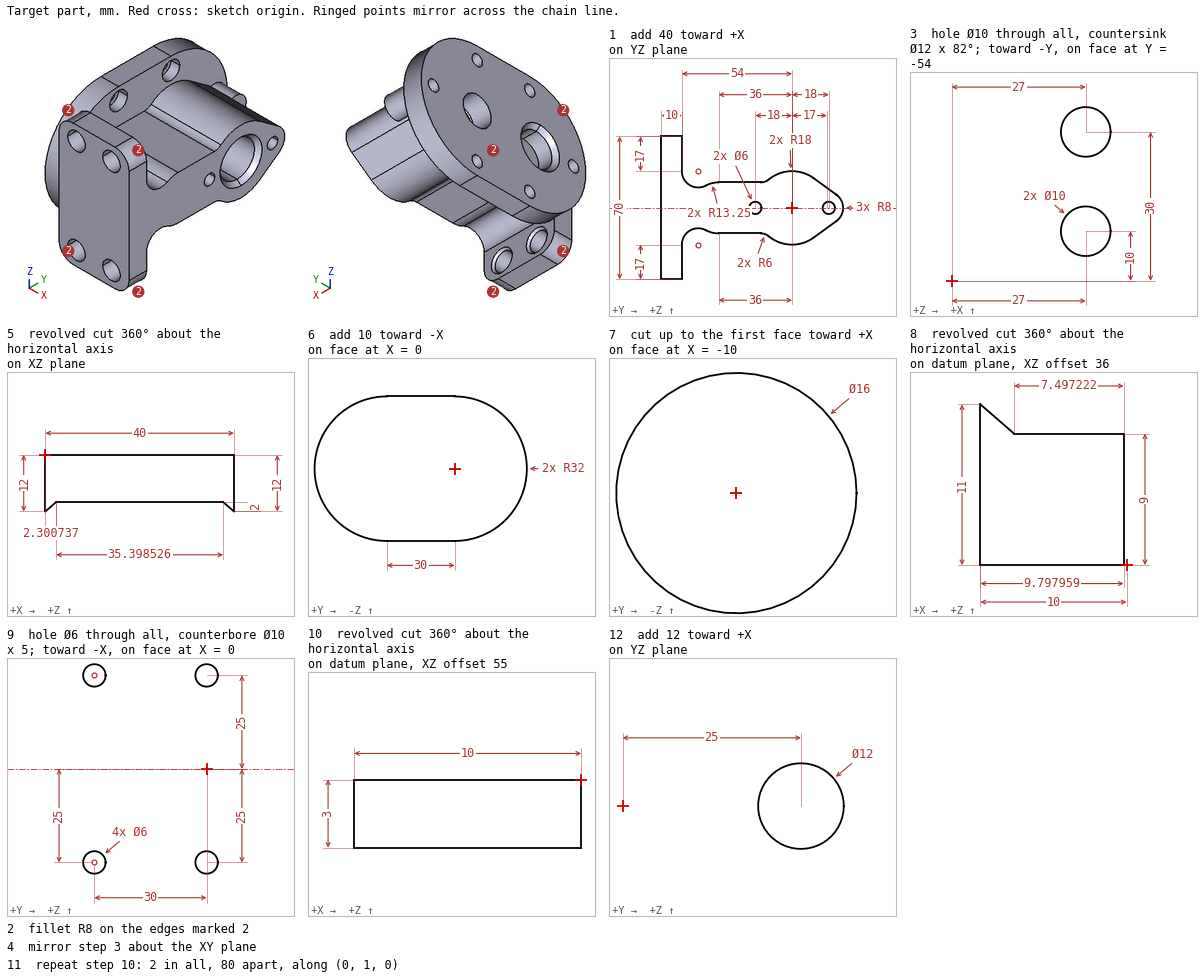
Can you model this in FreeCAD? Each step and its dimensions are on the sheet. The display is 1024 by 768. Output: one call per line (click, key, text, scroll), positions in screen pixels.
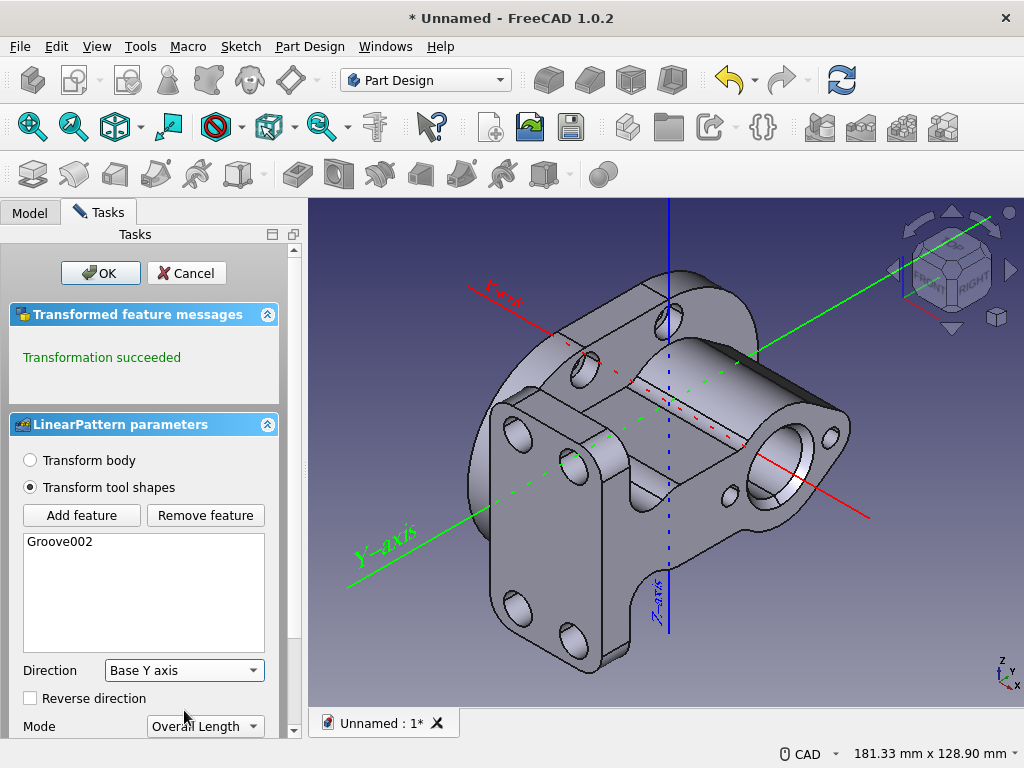
click(206, 726)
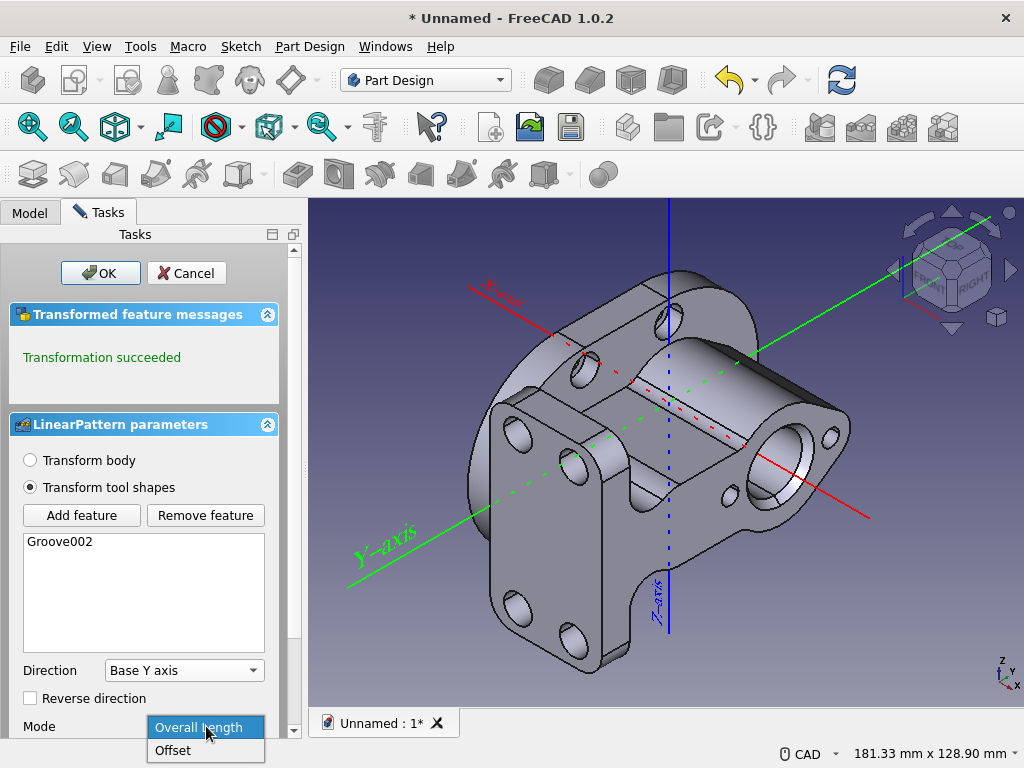
click(204, 750)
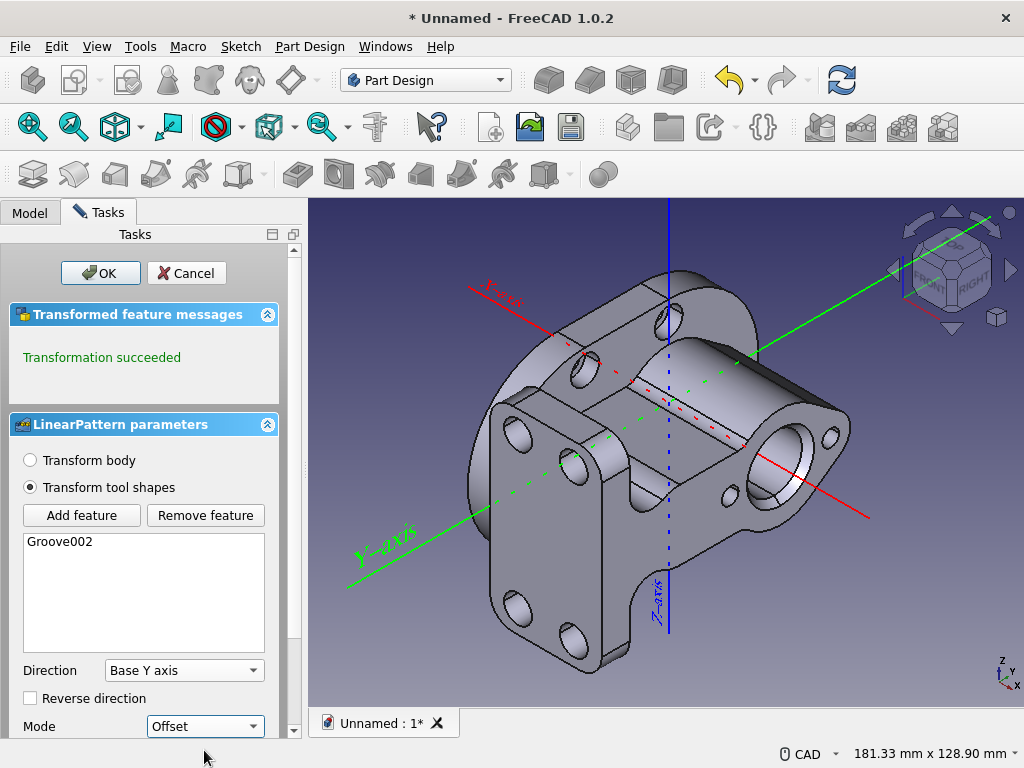
scroll(294, 491, down, 2)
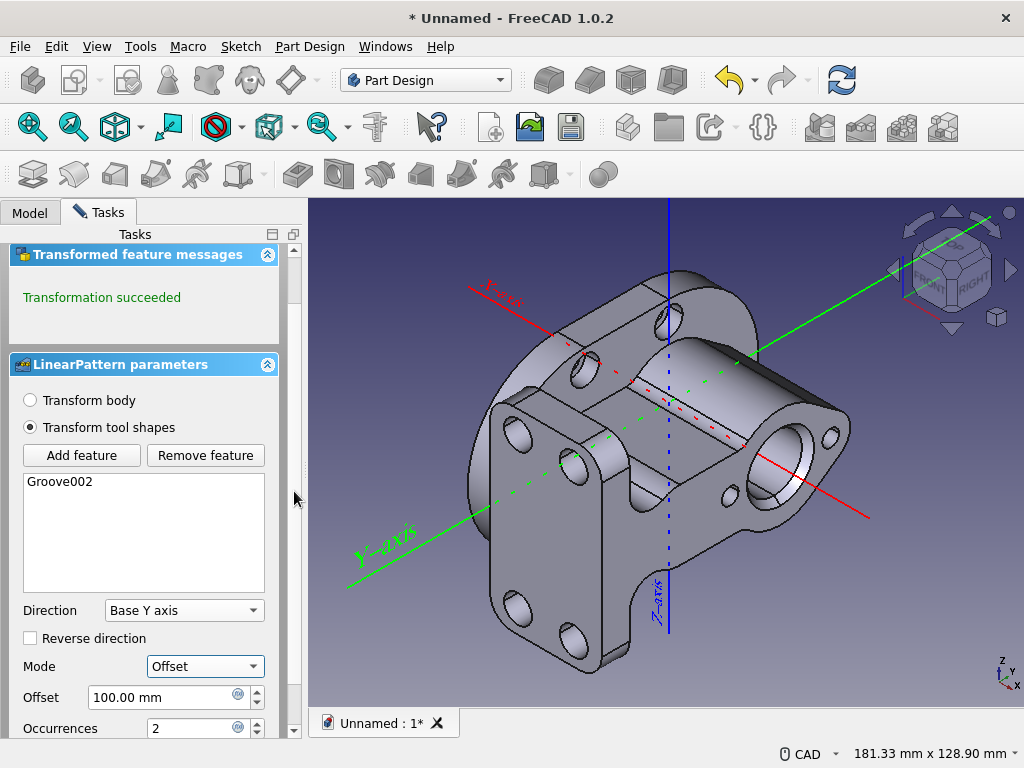
triple_click(170, 646)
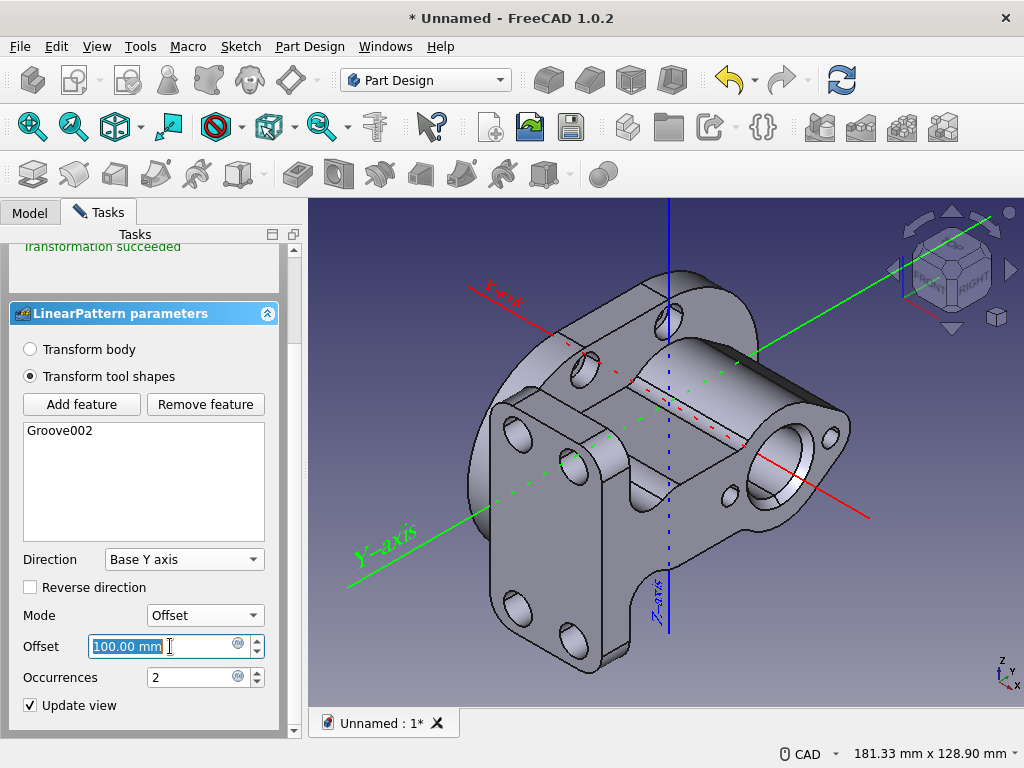
text(80)
key(Tab)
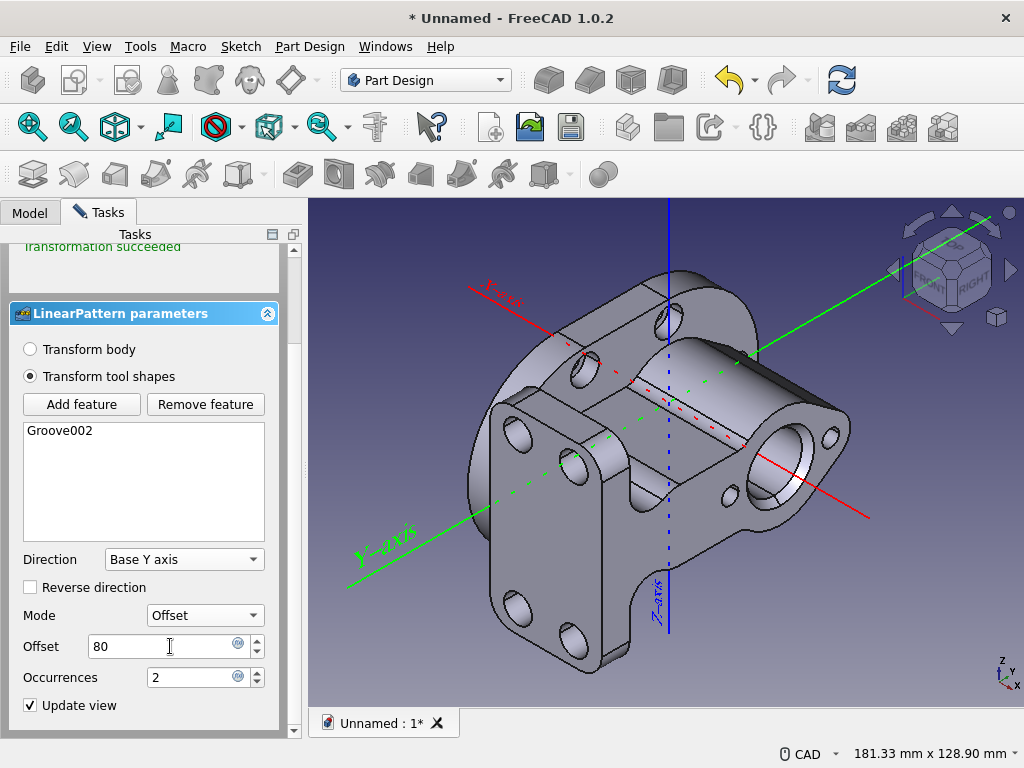
triple_click(199, 678)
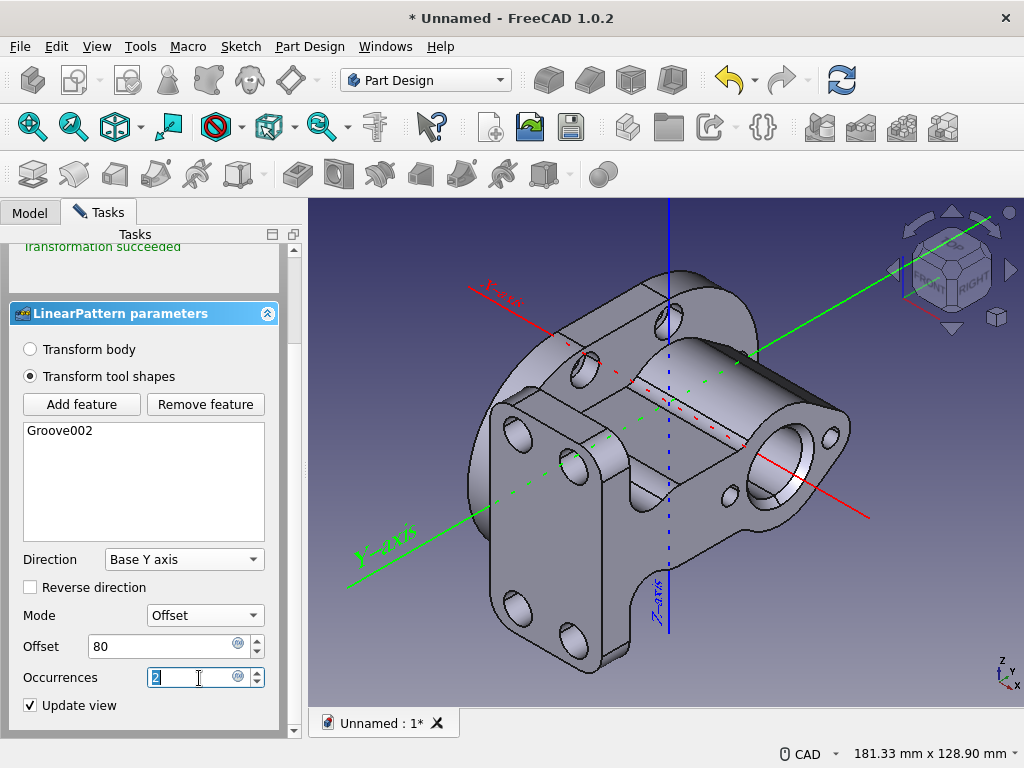
text(2)
key(Tab)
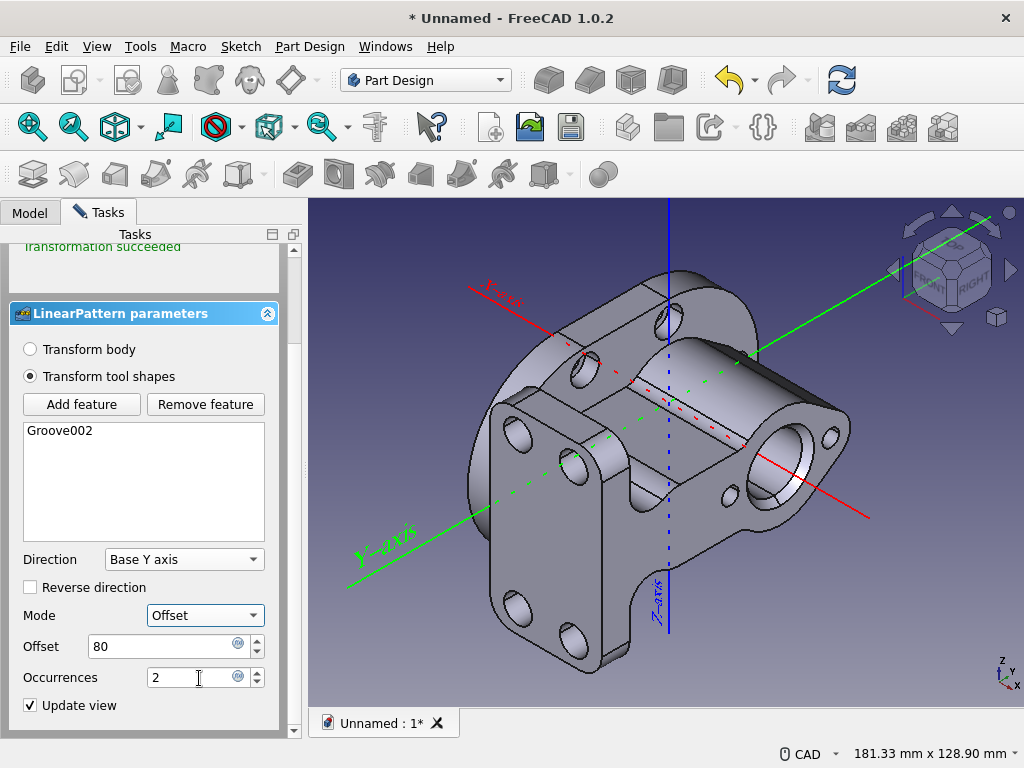
scroll(294, 491, up, 3)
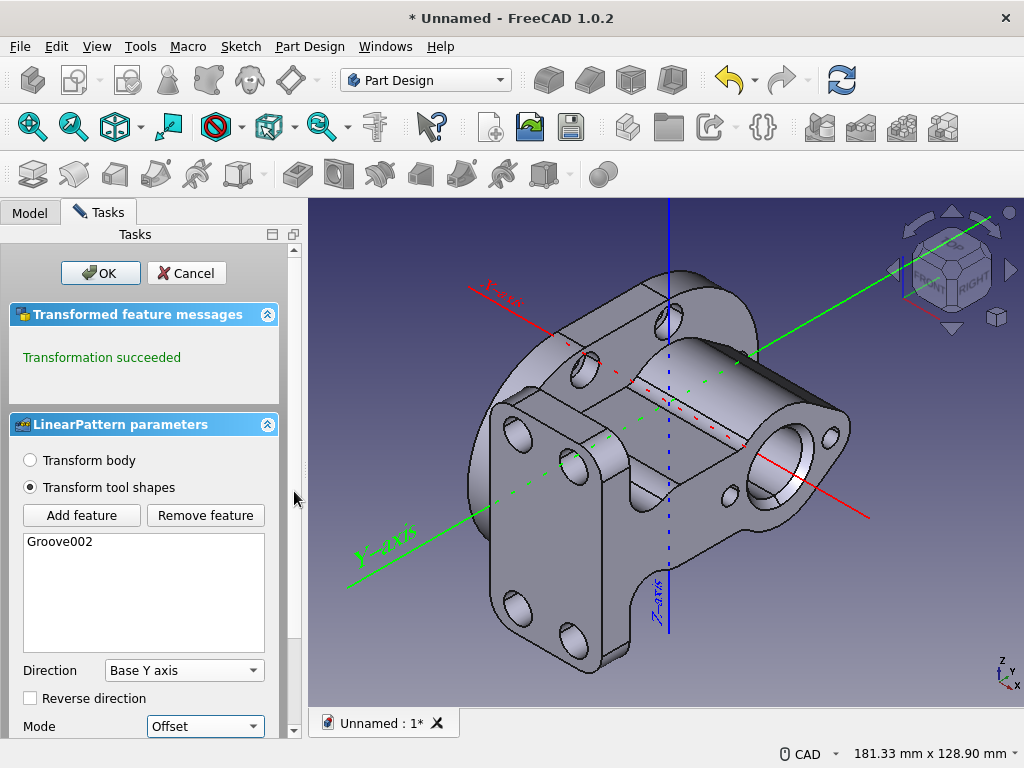
click(101, 273)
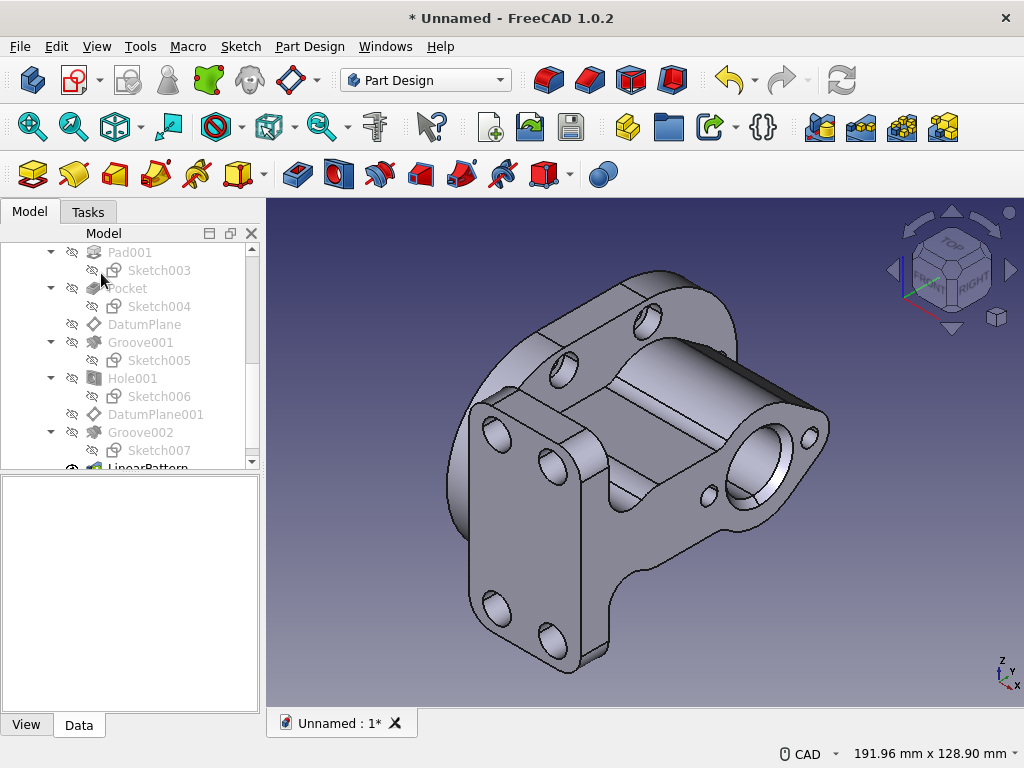
click(74, 80)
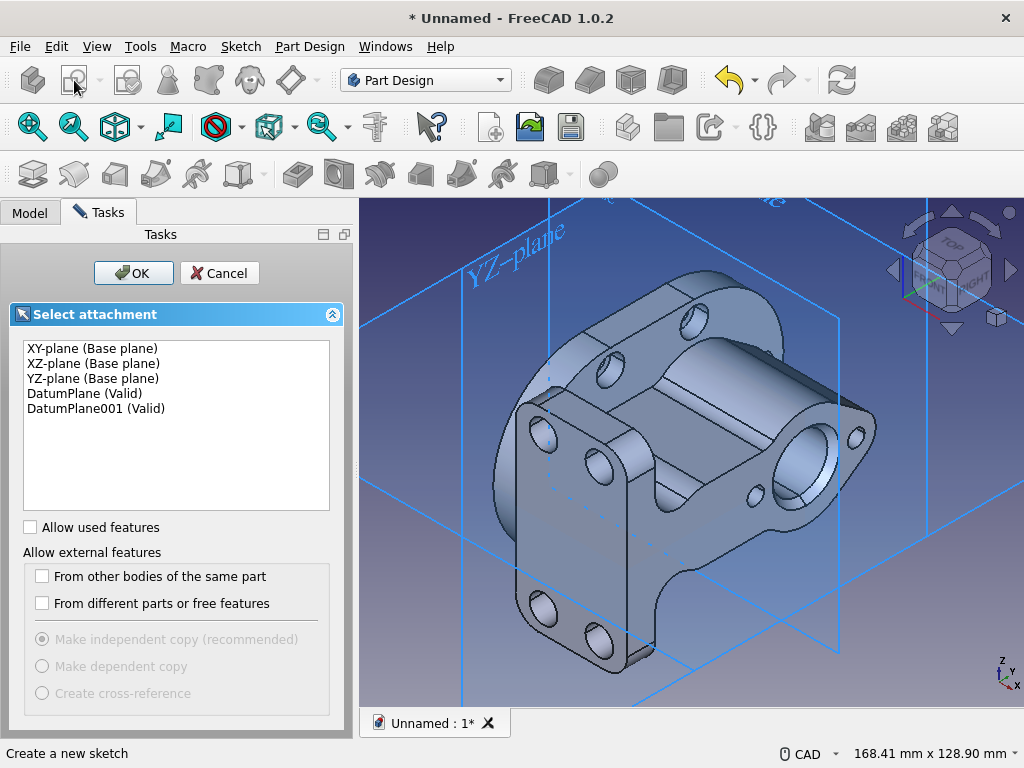
click(84, 378)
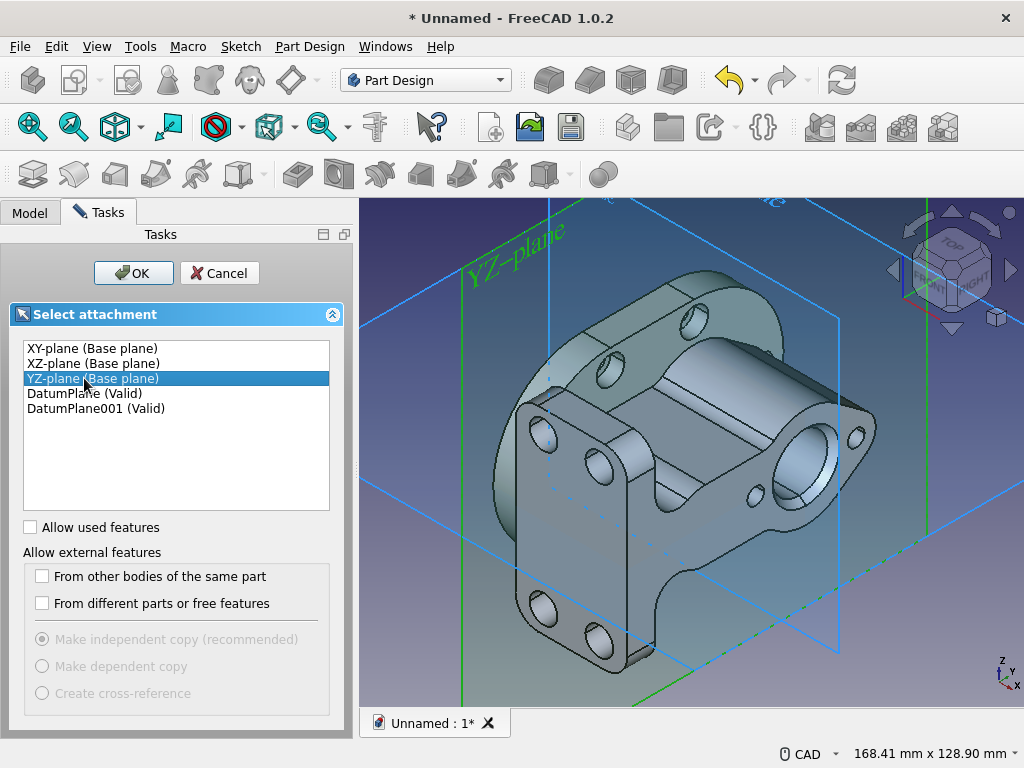
click(134, 273)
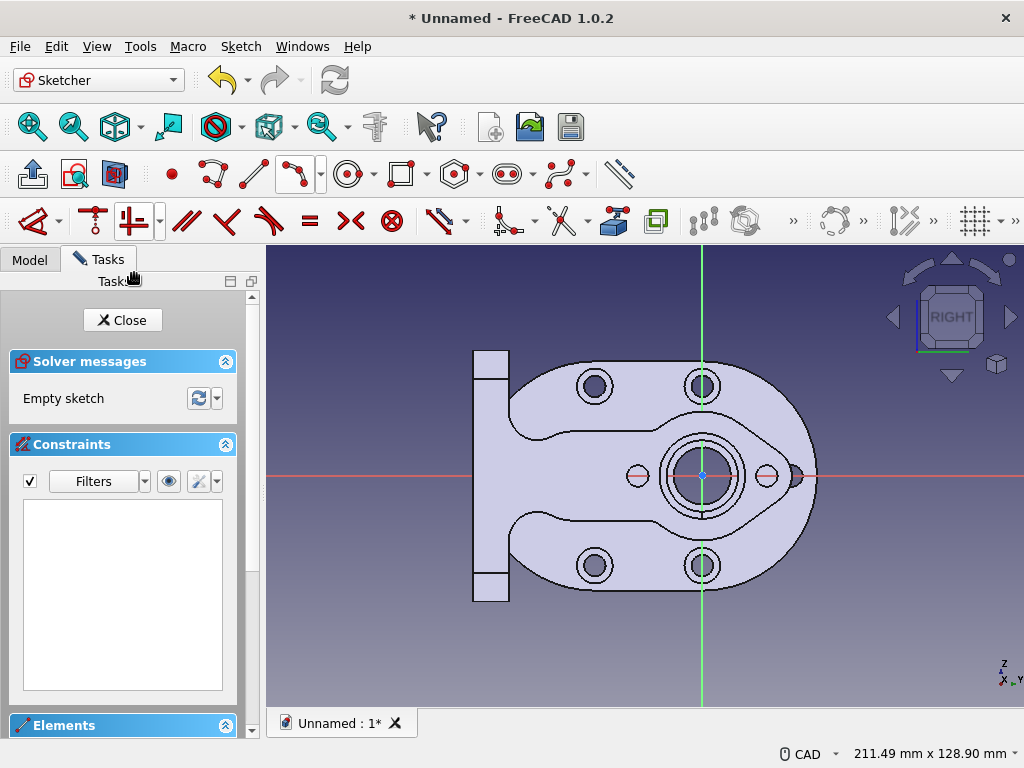
click(115, 174)